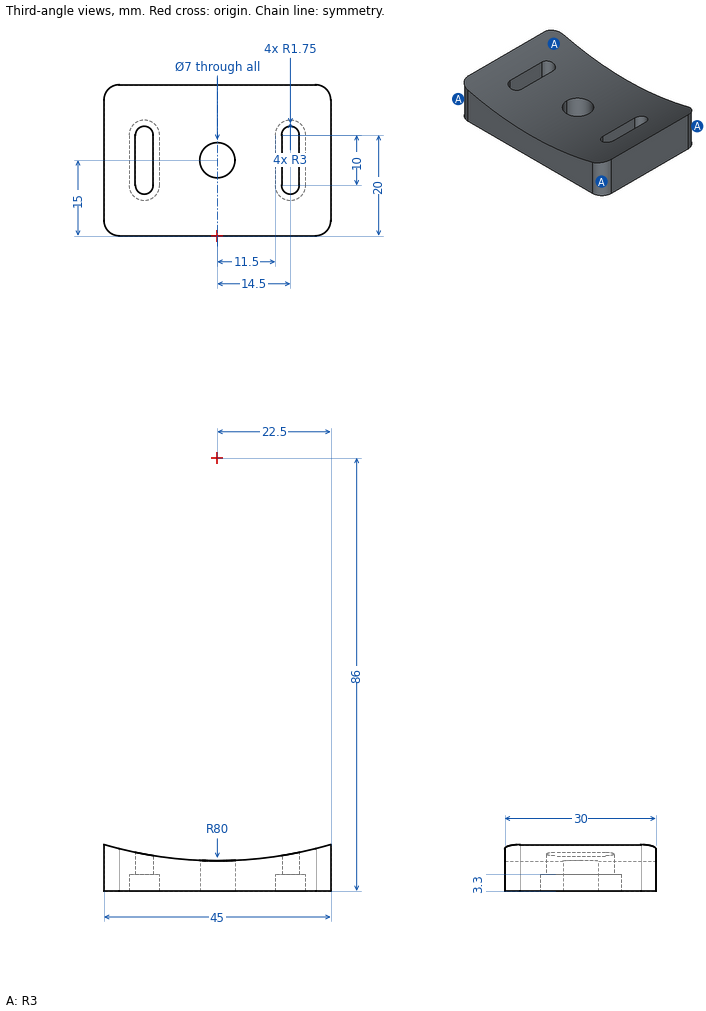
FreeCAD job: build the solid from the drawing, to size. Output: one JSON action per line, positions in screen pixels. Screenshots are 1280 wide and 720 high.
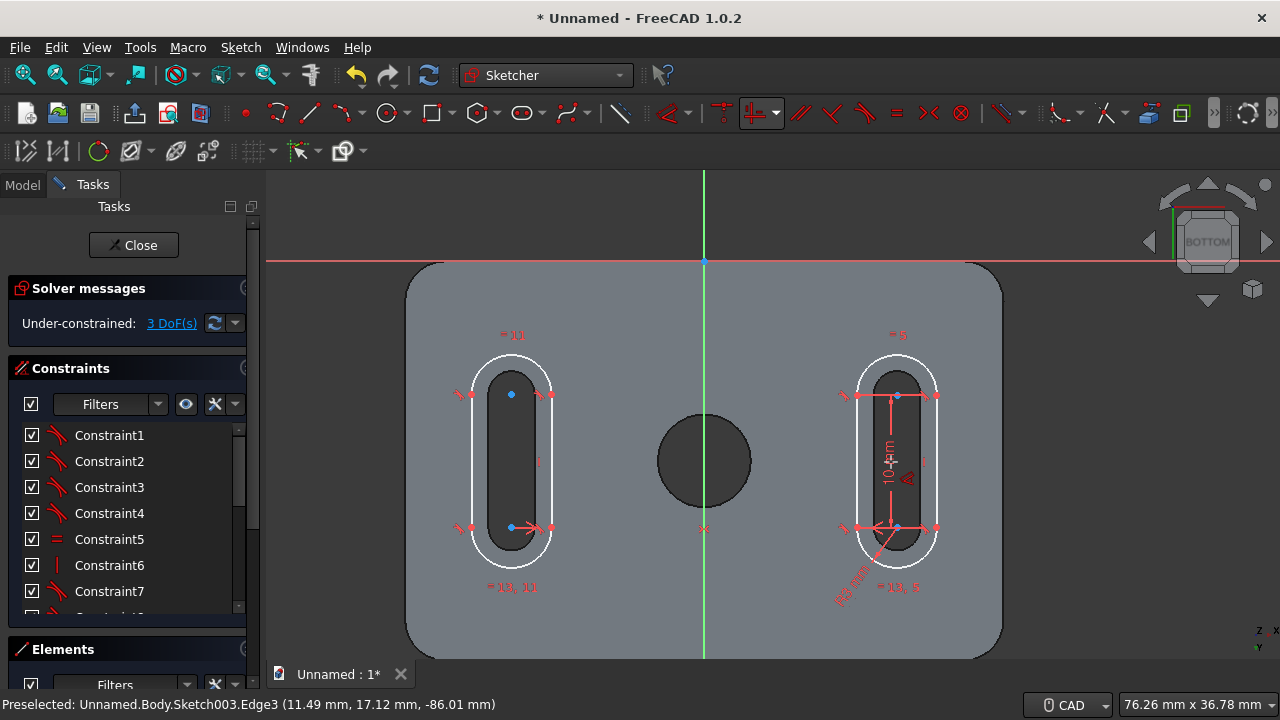
{"action": "left_click", "coordinate": [472, 488]}
{"action": "left_click", "coordinate": [438, 461]}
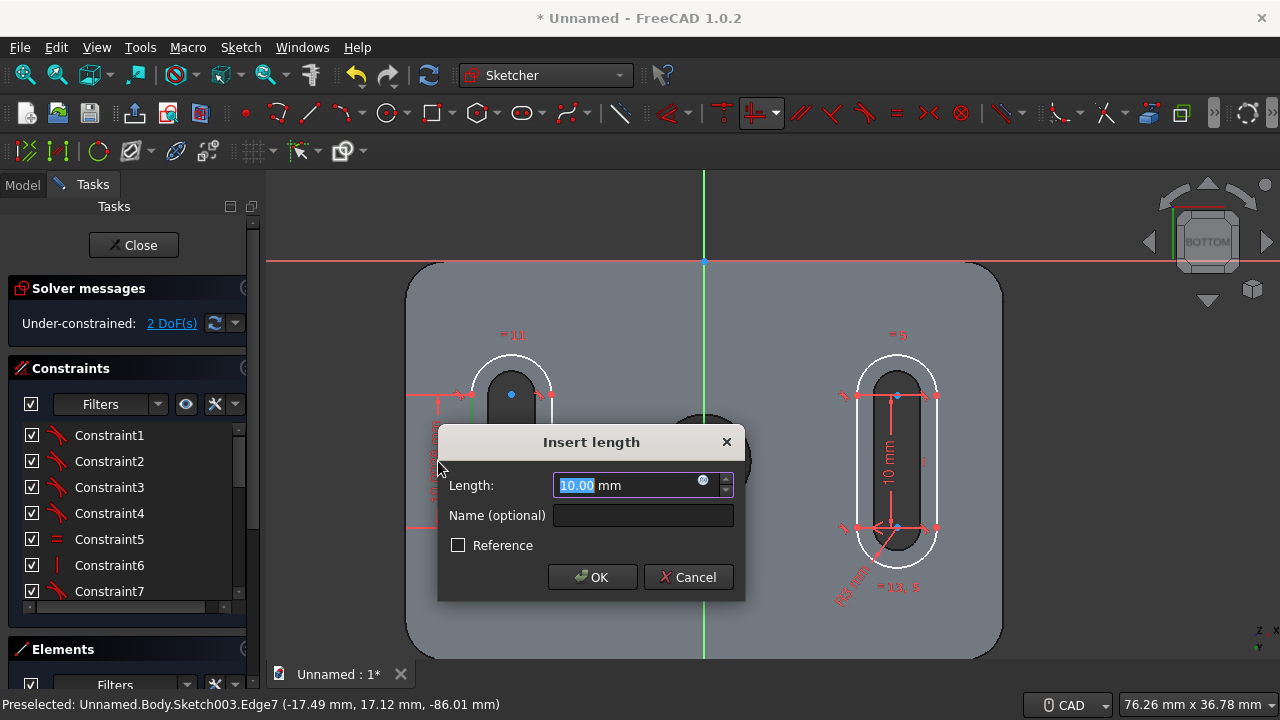
{"action": "type", "text": "10"}
{"action": "key", "text": "Return"}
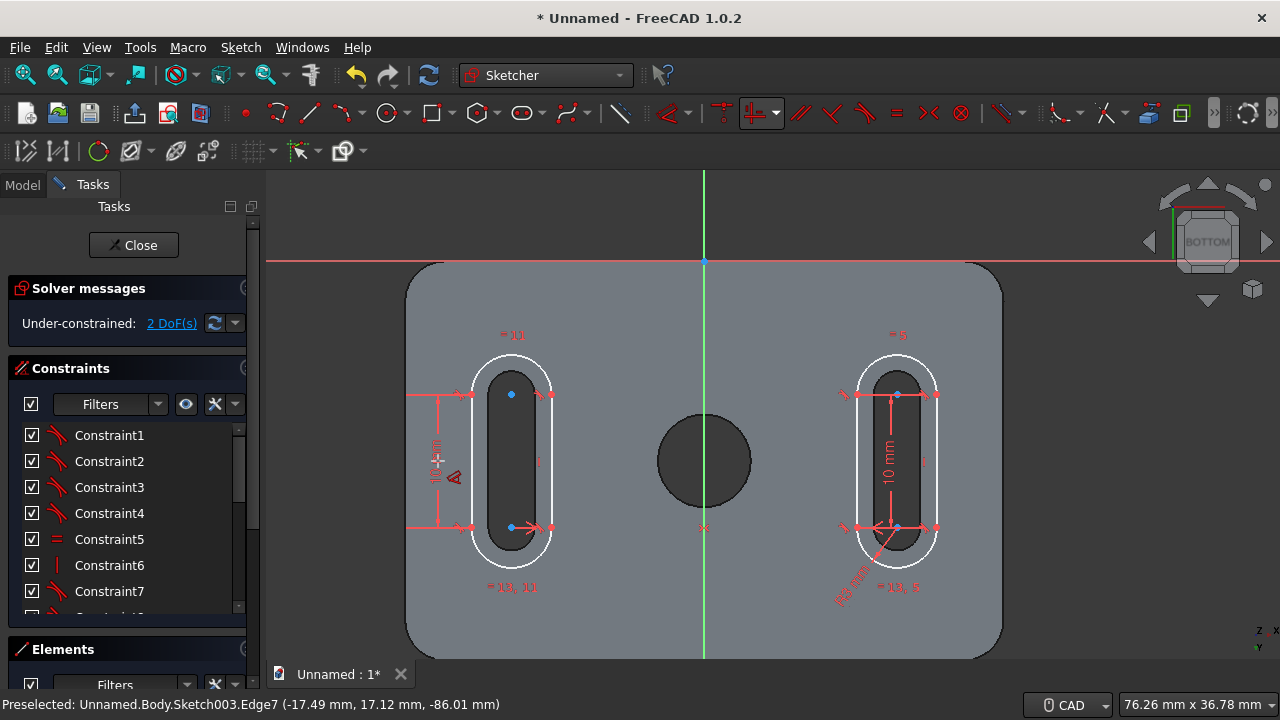
{"action": "left_click", "coordinate": [857, 528]}
{"action": "left_click", "coordinate": [891, 395]}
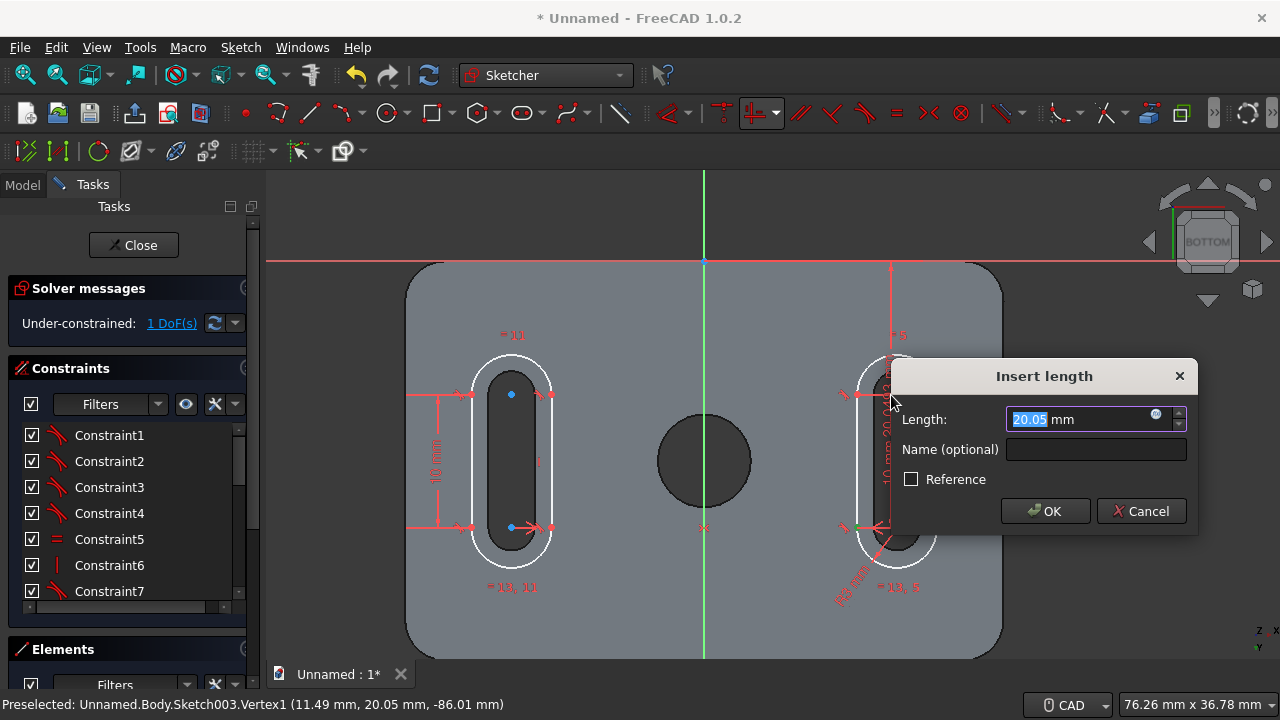
{"action": "type", "text": "20"}
{"action": "key", "text": "Return"}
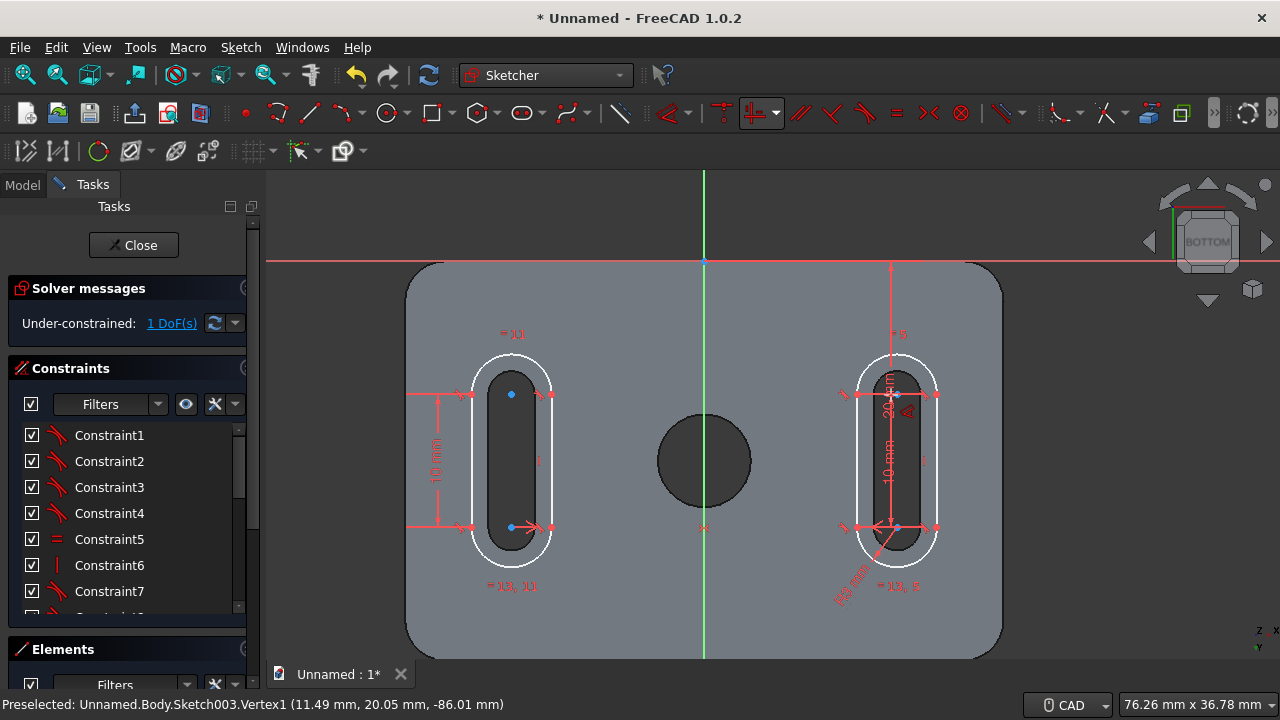
{"action": "left_click", "coordinate": [857, 527]}
{"action": "left_click", "coordinate": [781, 227]}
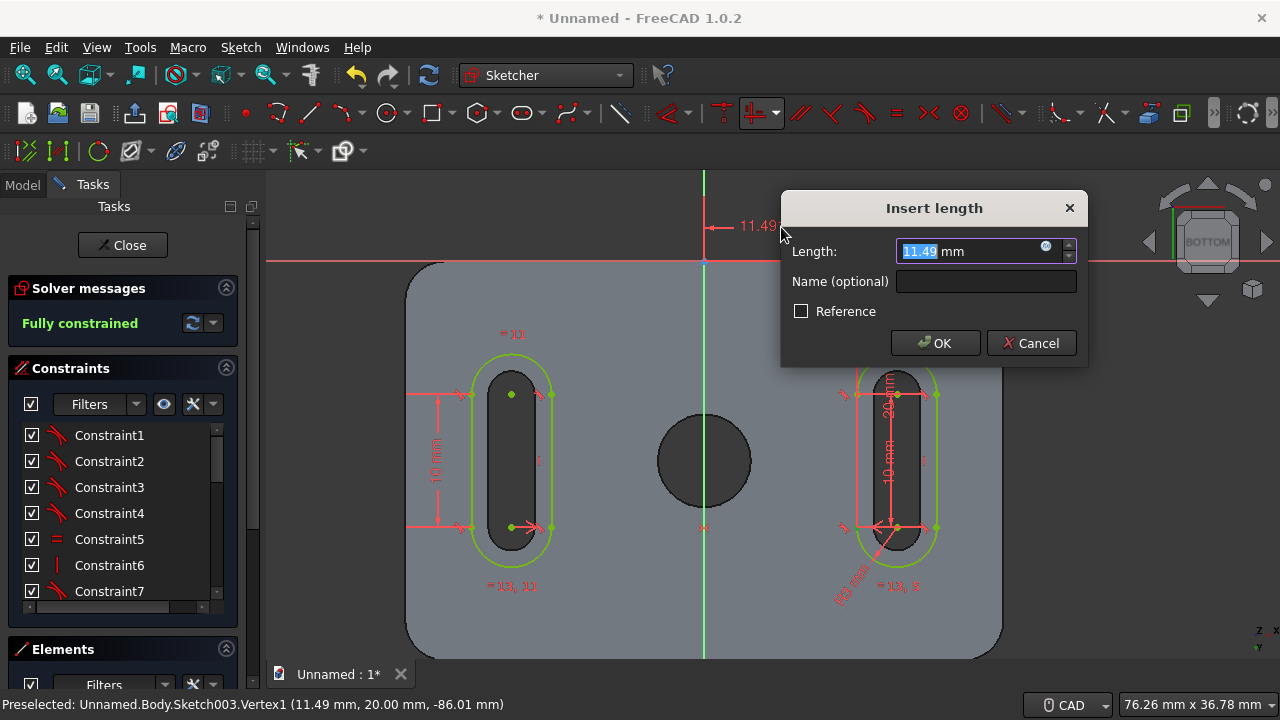
{"action": "type", "text": "11.5"}
{"action": "key", "text": "Return"}
{"action": "key", "text": "Escape"}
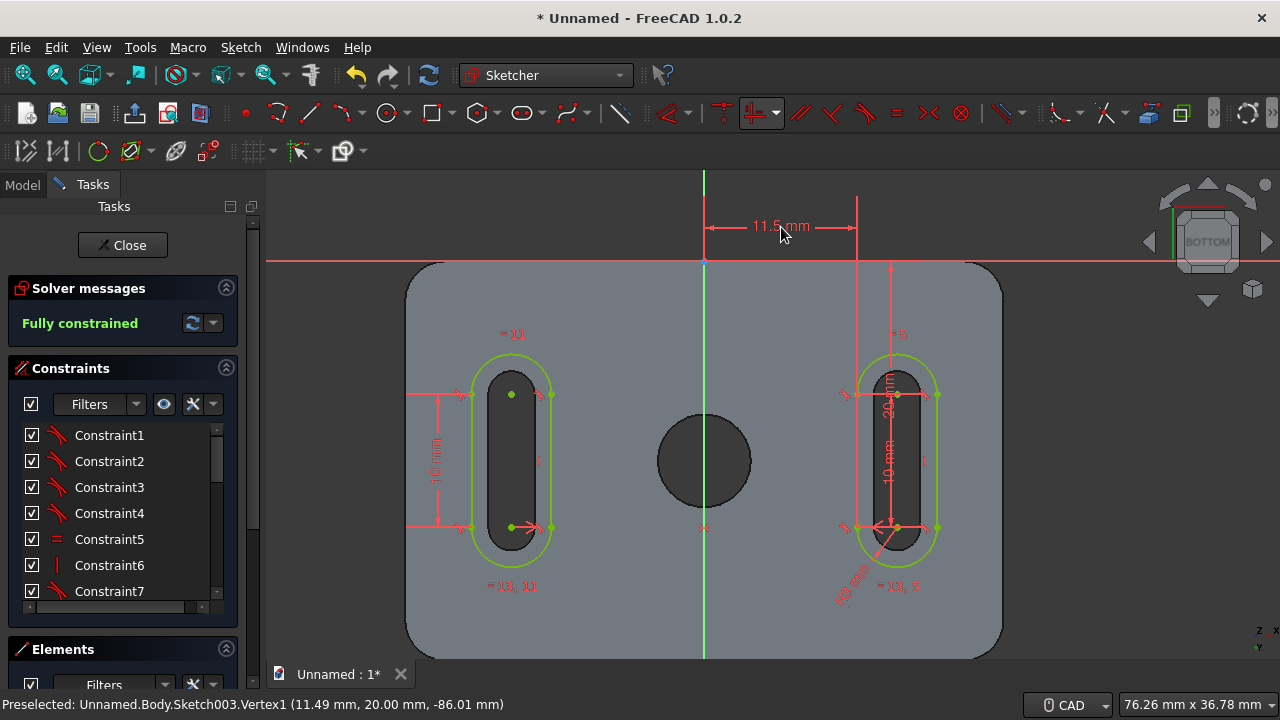
{"action": "left_click", "coordinate": [123, 245]}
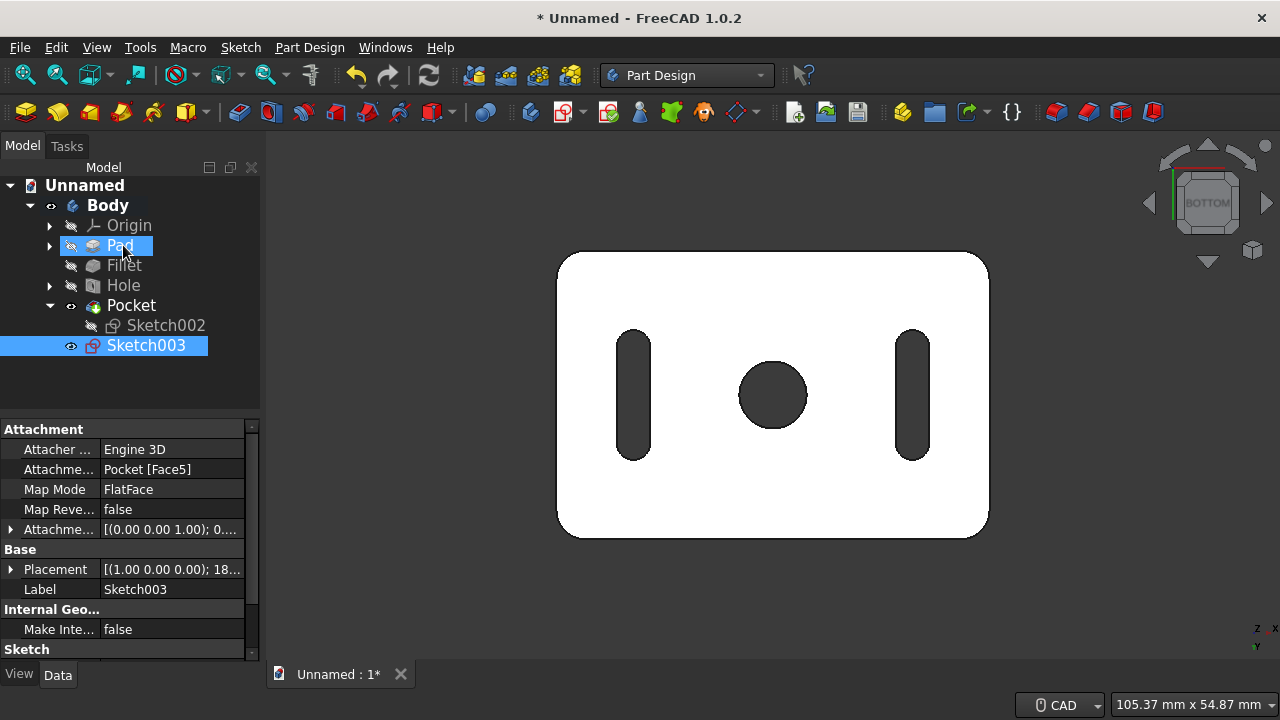
{"action": "left_click", "coordinate": [240, 112]}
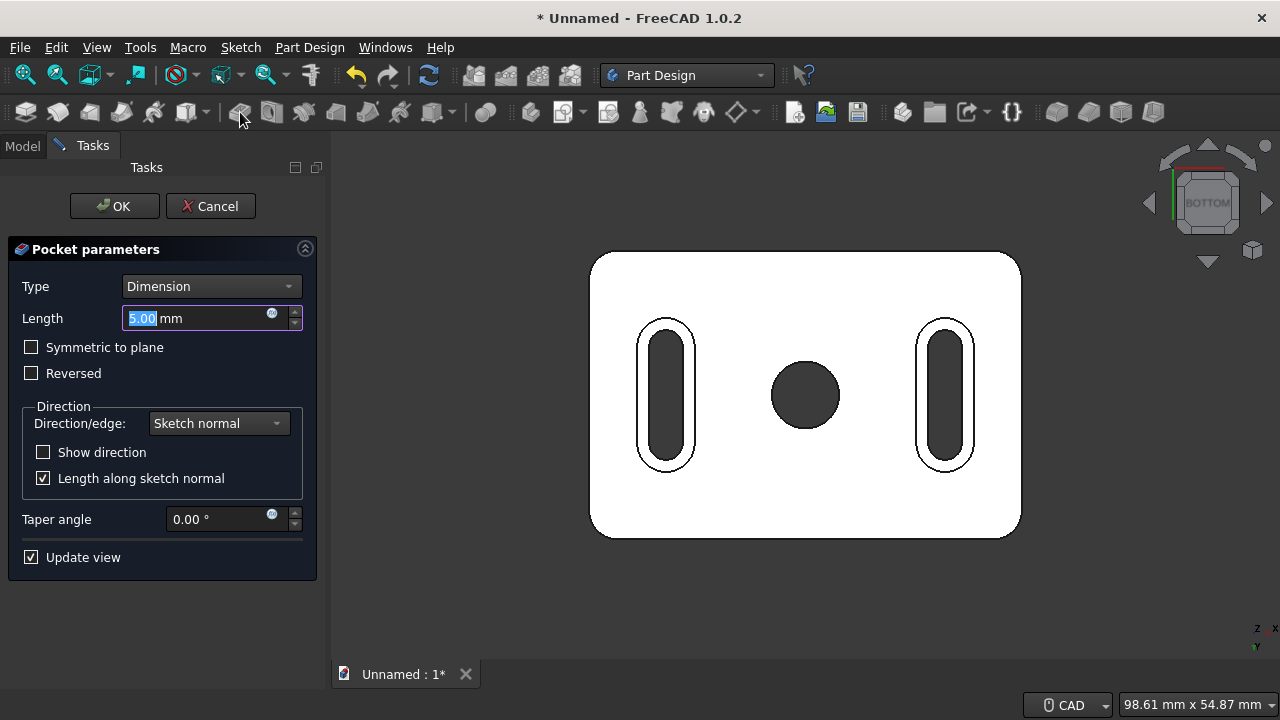
{"action": "type", "text": "3.3"}
{"action": "key", "text": "Tab"}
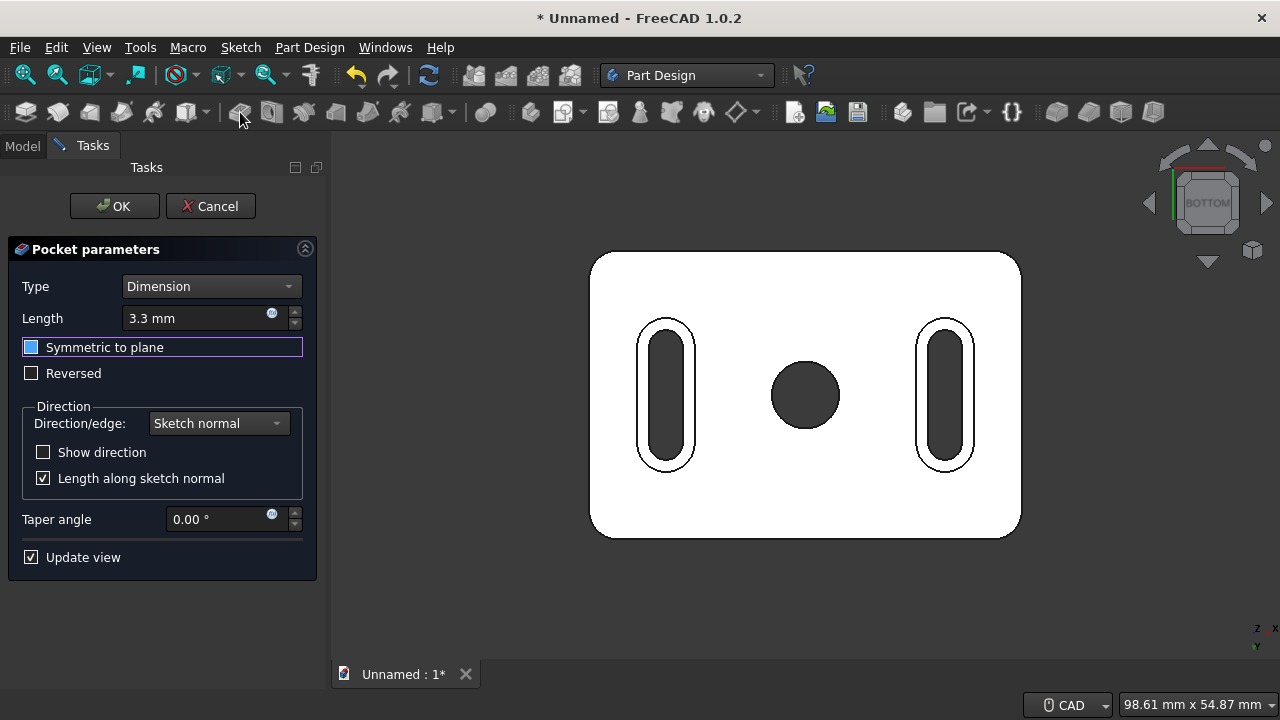
{"action": "left_click", "coordinate": [115, 206]}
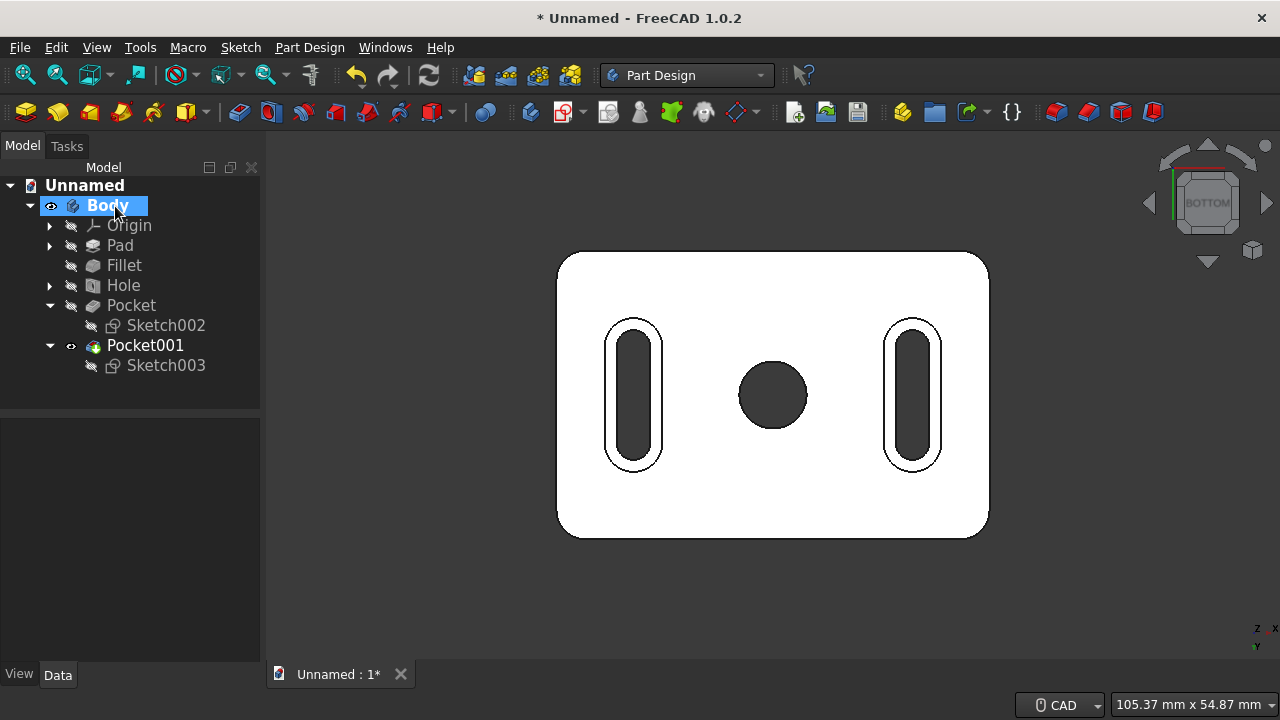
{"action": "key", "text": "0"}